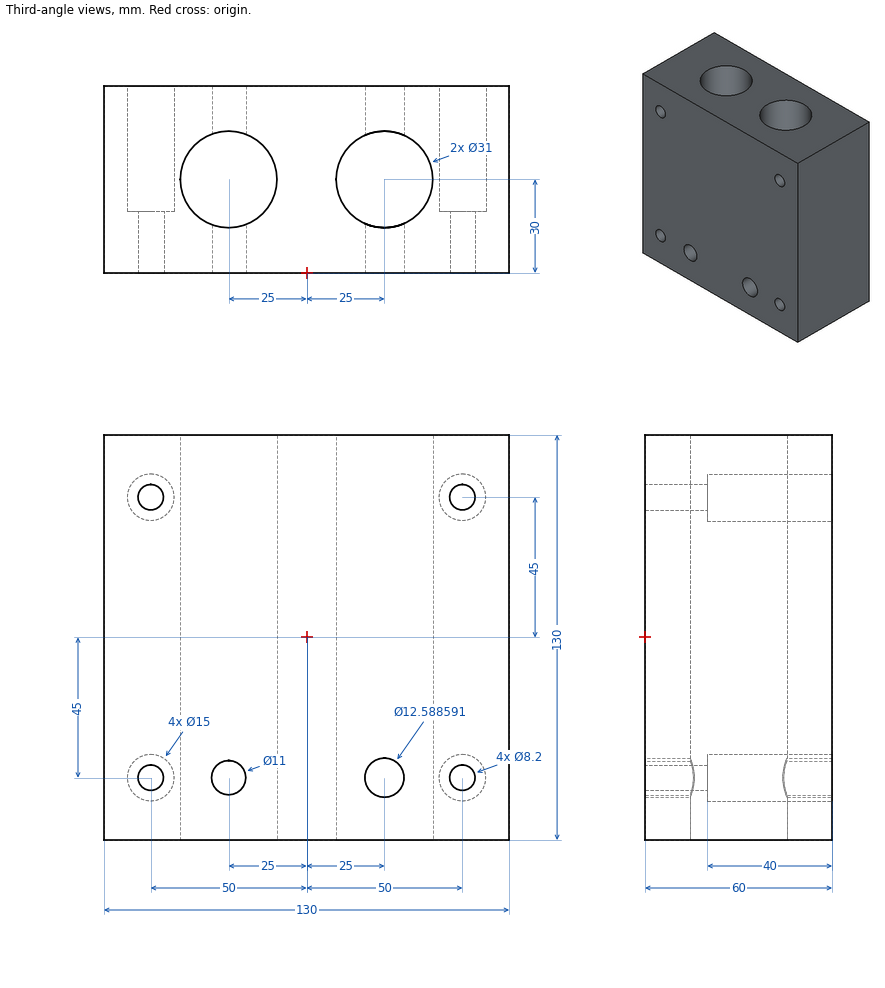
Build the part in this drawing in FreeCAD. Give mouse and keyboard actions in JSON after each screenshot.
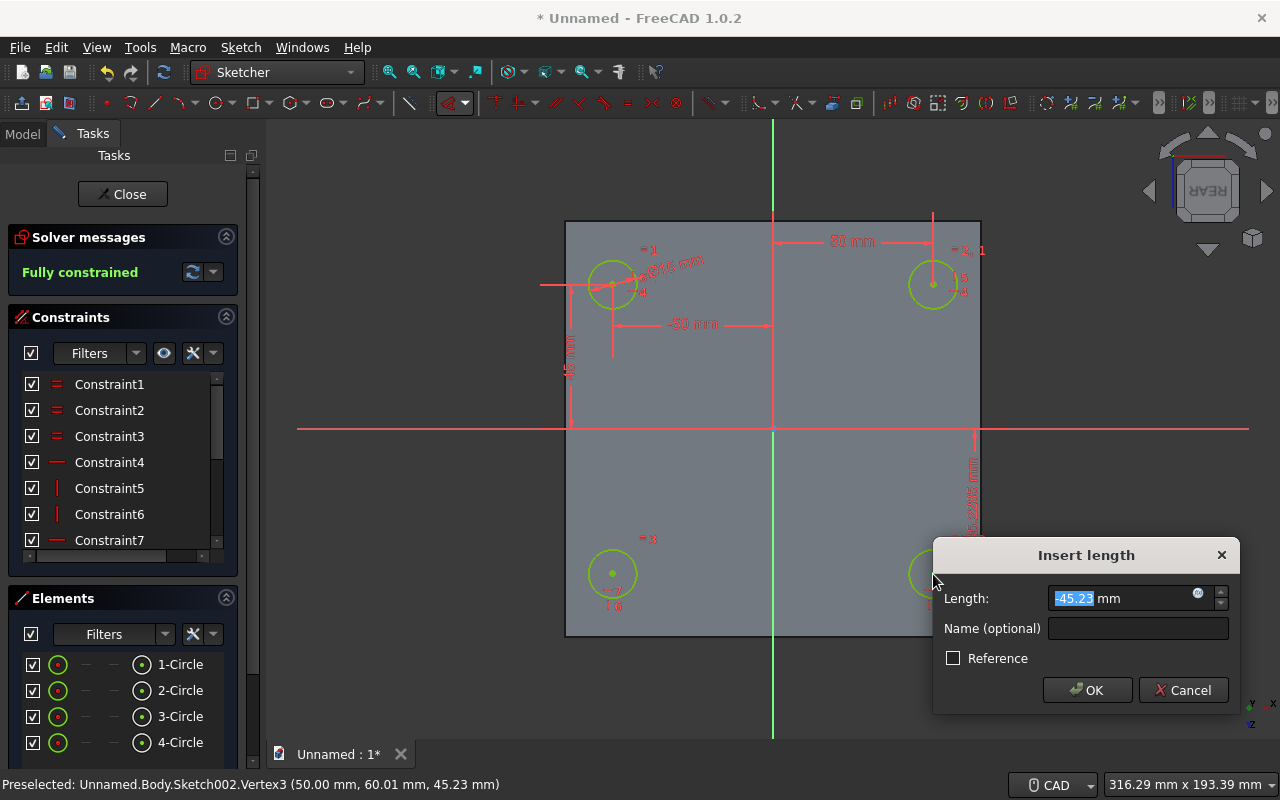
{"action": "type", "text": "-45"}
{"action": "key", "text": "Return"}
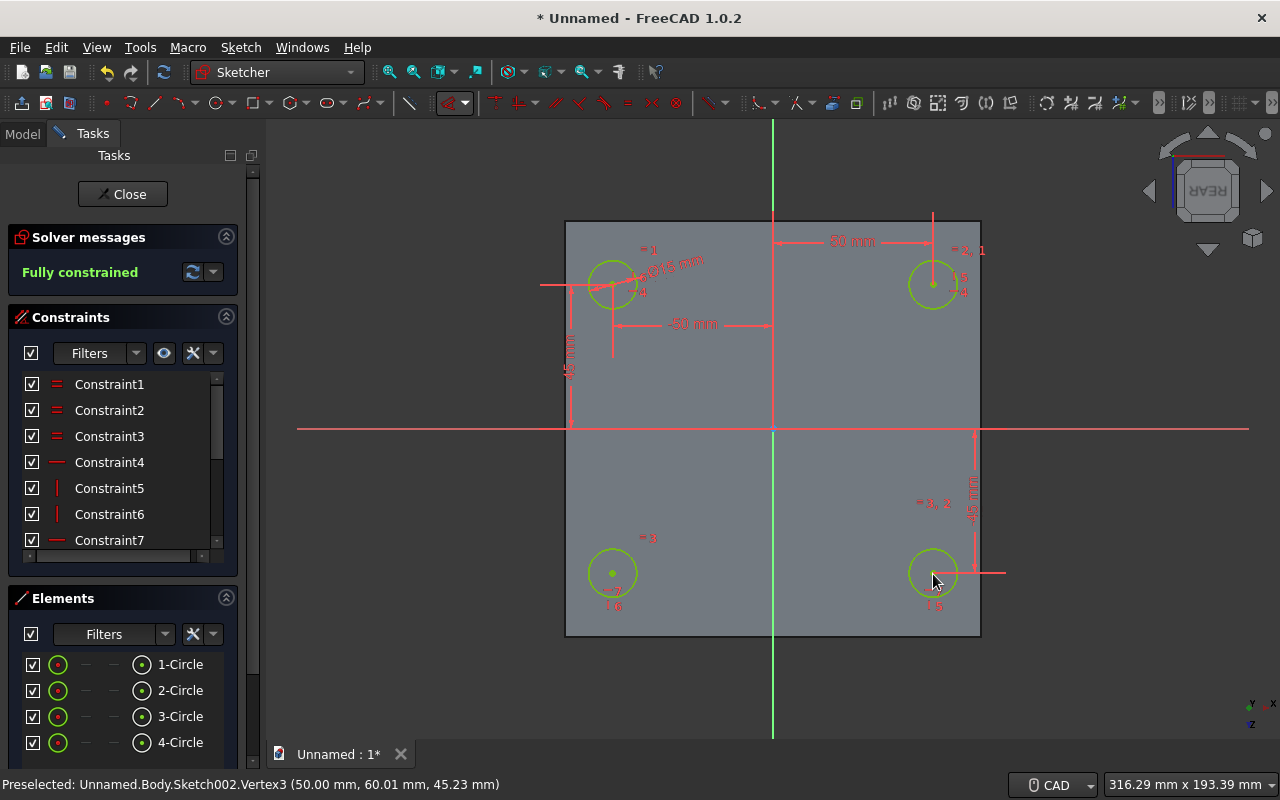
{"action": "left_click", "coordinate": [123, 194]}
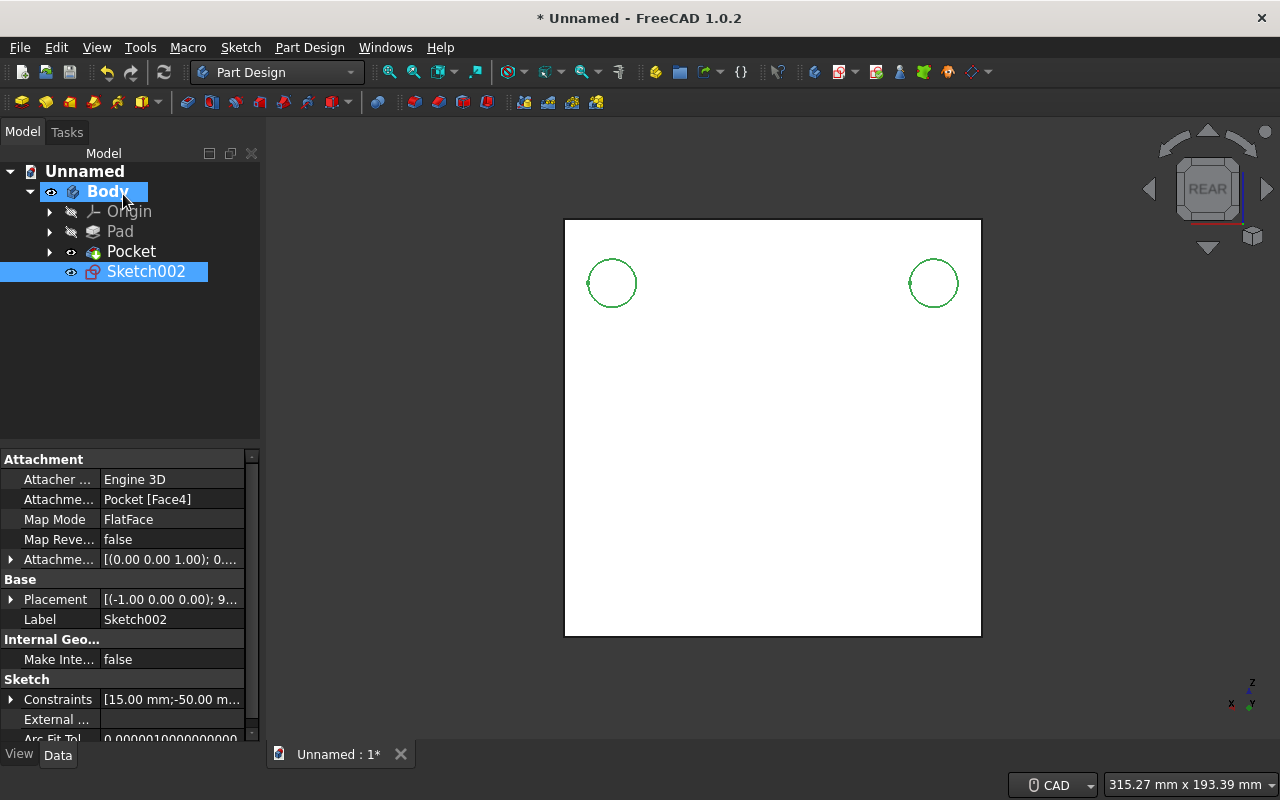
{"action": "left_click", "coordinate": [188, 102]}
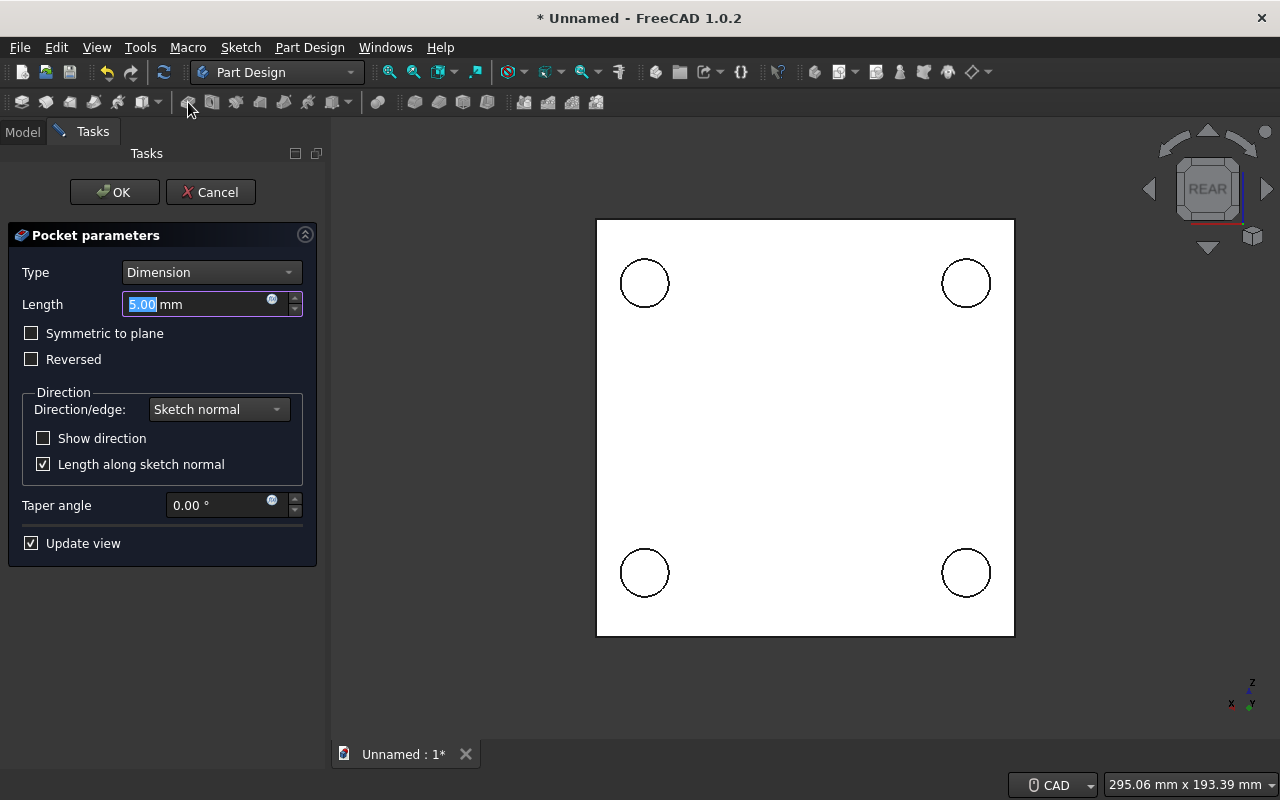
{"action": "type", "text": "40"}
{"action": "key", "text": "Tab"}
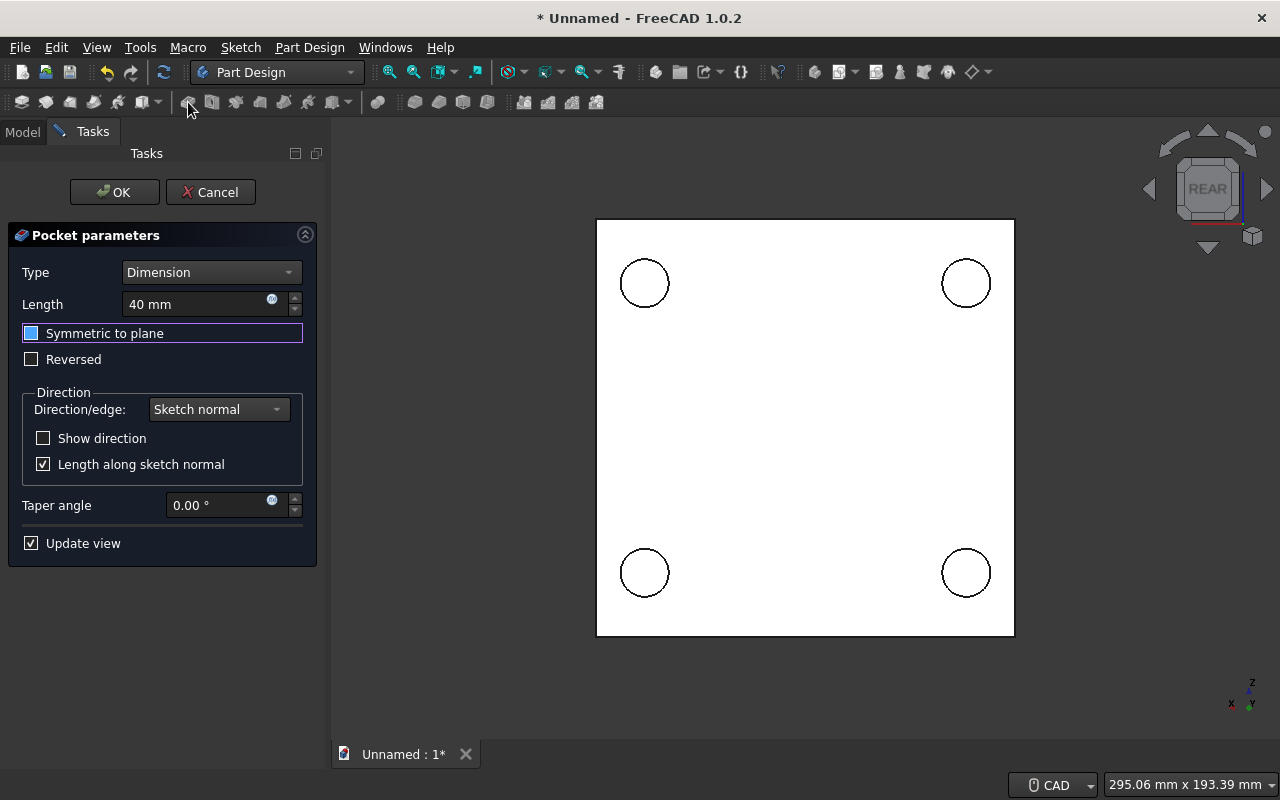
{"action": "left_click", "coordinate": [115, 192]}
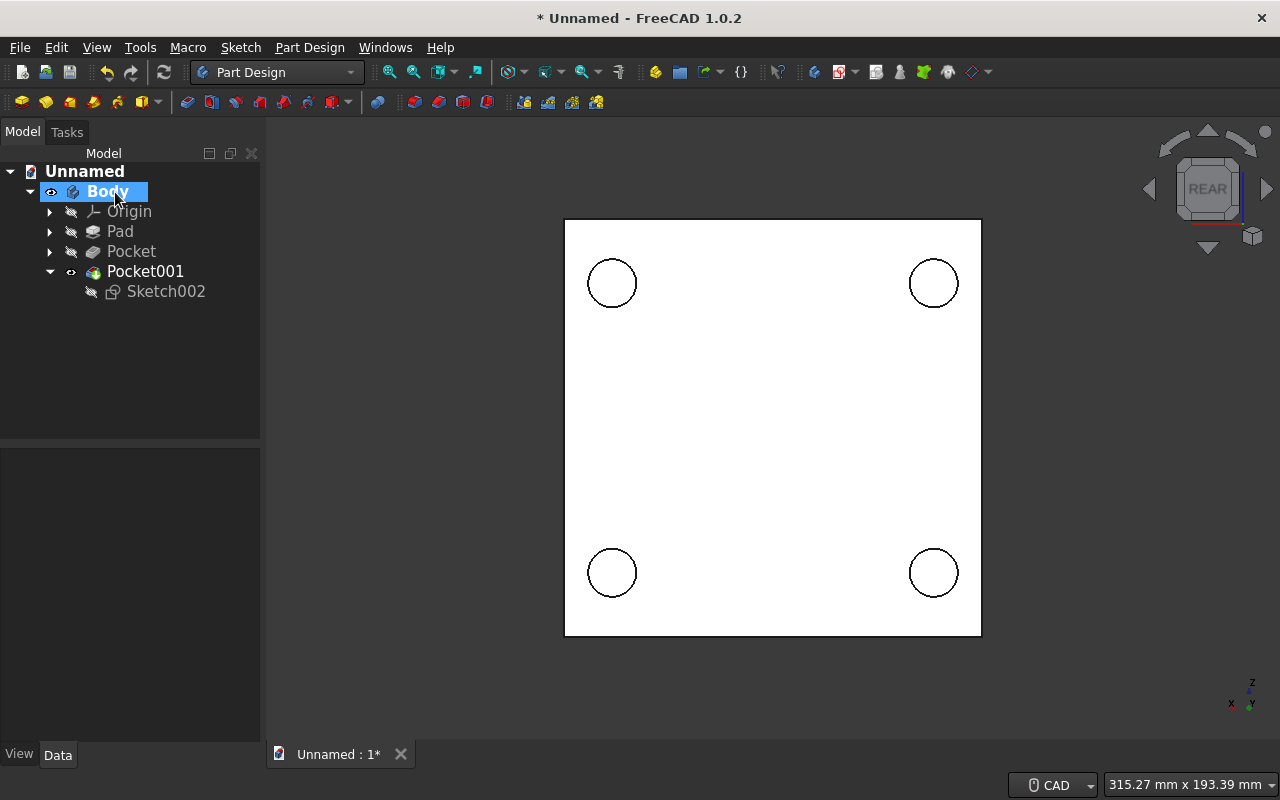
{"action": "left_click", "coordinate": [612, 282]}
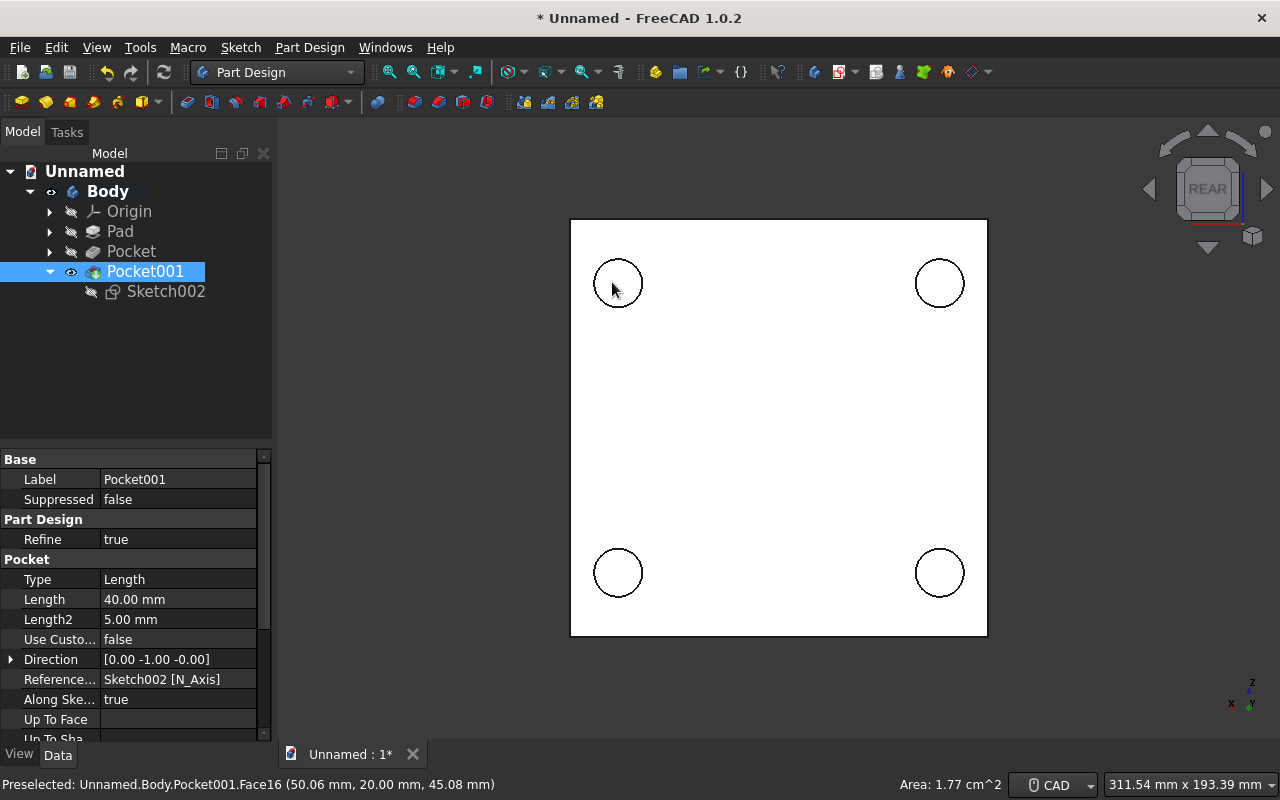
{"action": "left_click", "coordinate": [840, 72]}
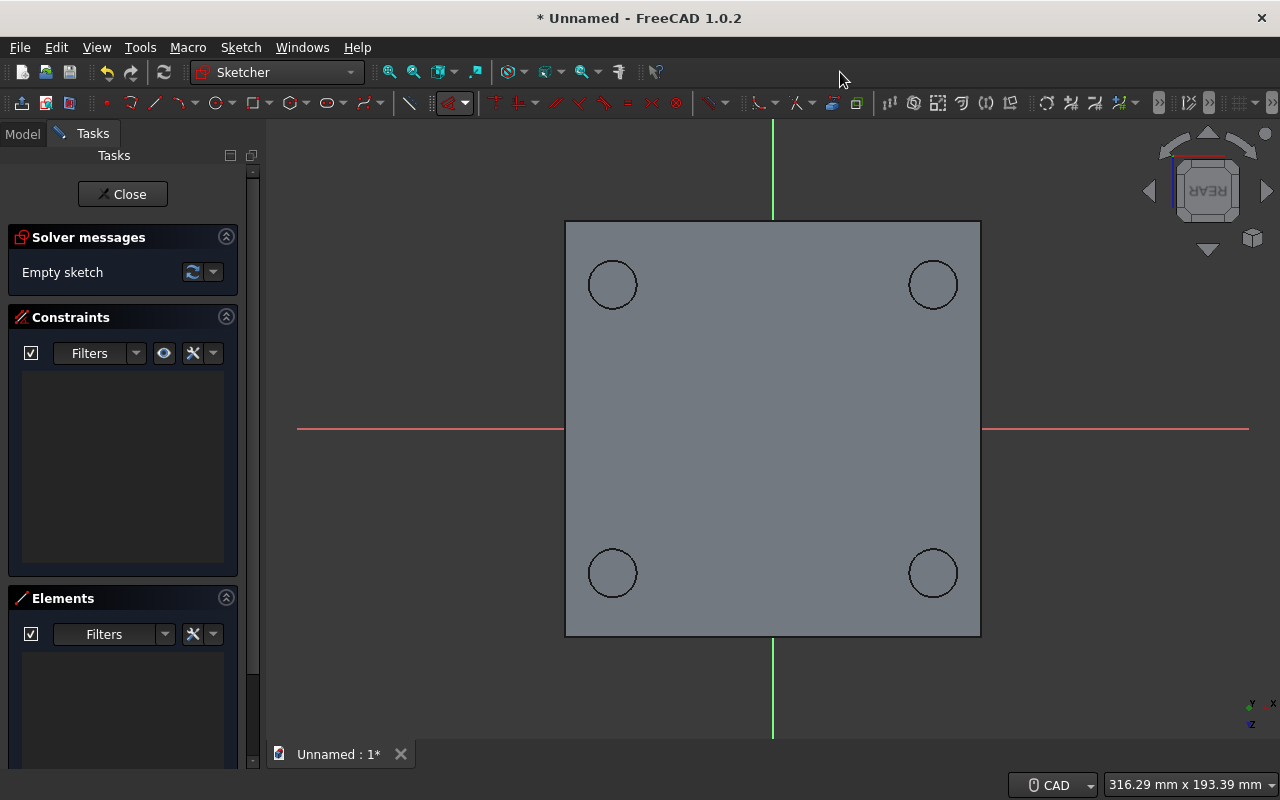
{"action": "key", "text": "g c"}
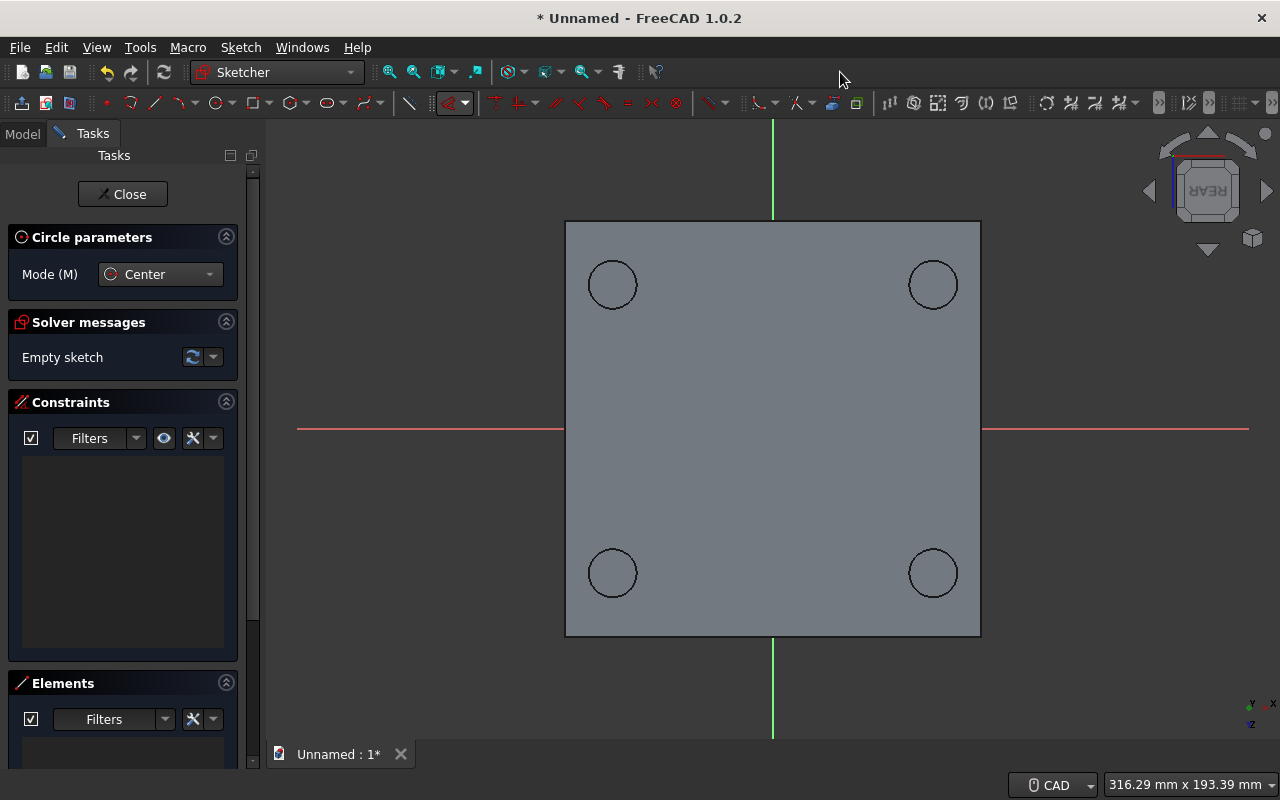
{"action": "scroll", "coordinate": [933, 285], "scroll_direction": "up", "scroll_amount": 3}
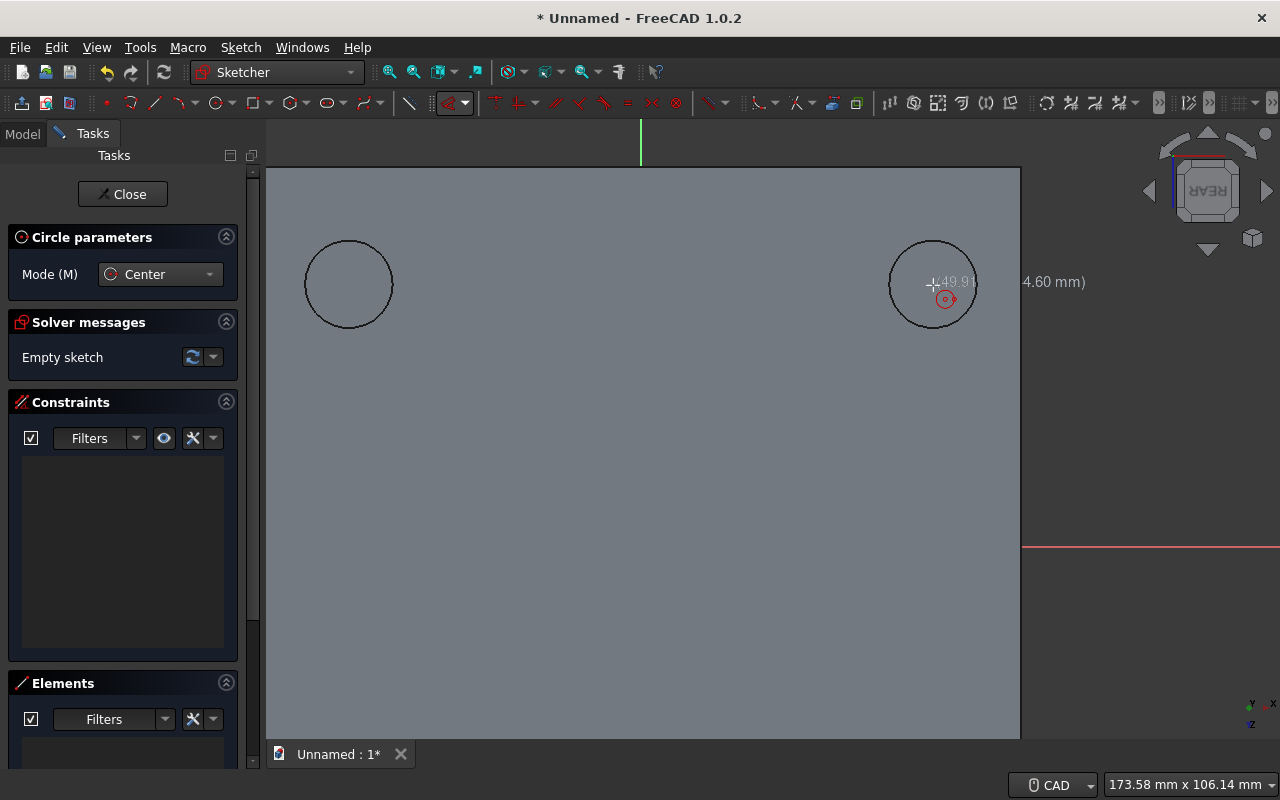
{"action": "left_click", "coordinate": [933, 284]}
{"action": "left_click", "coordinate": [950, 267]}